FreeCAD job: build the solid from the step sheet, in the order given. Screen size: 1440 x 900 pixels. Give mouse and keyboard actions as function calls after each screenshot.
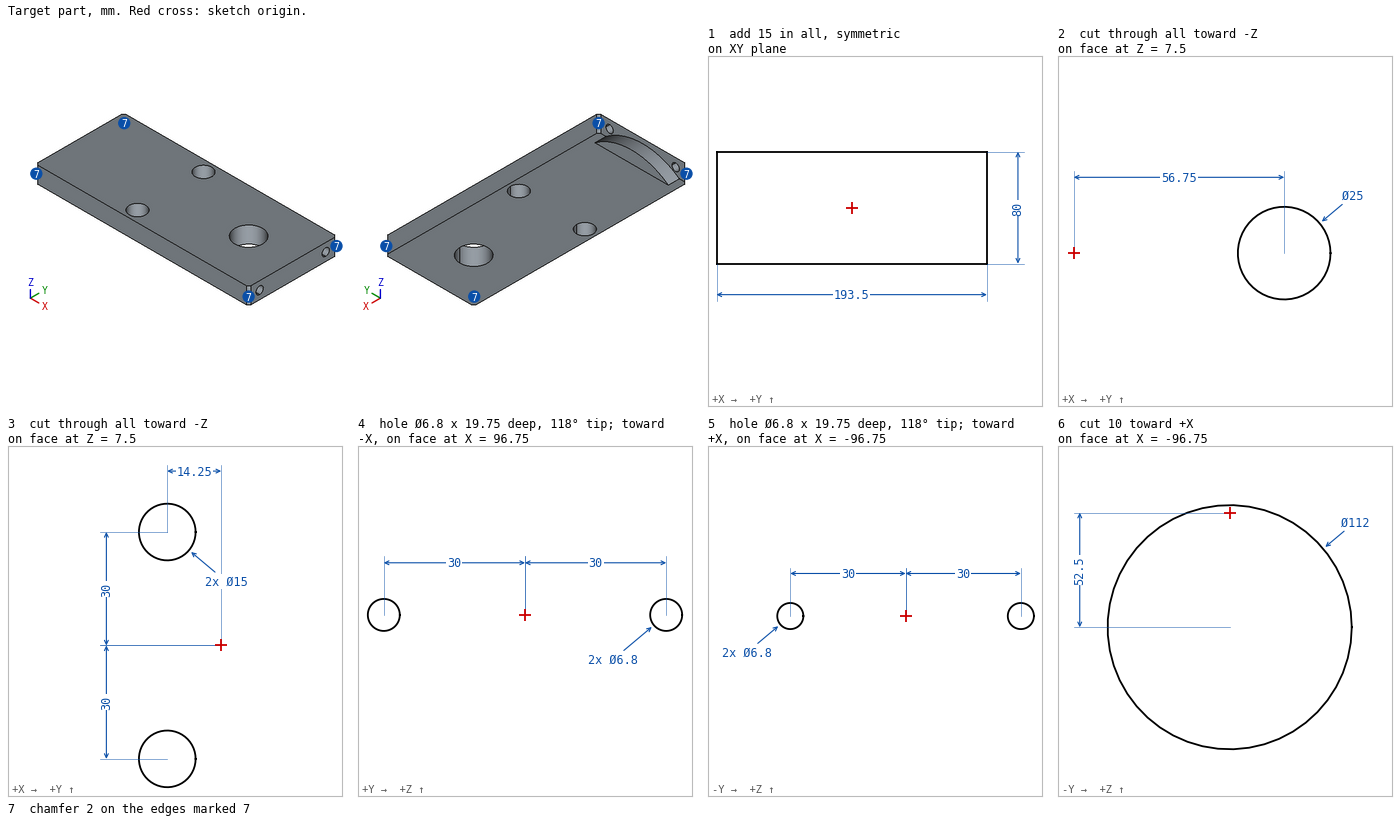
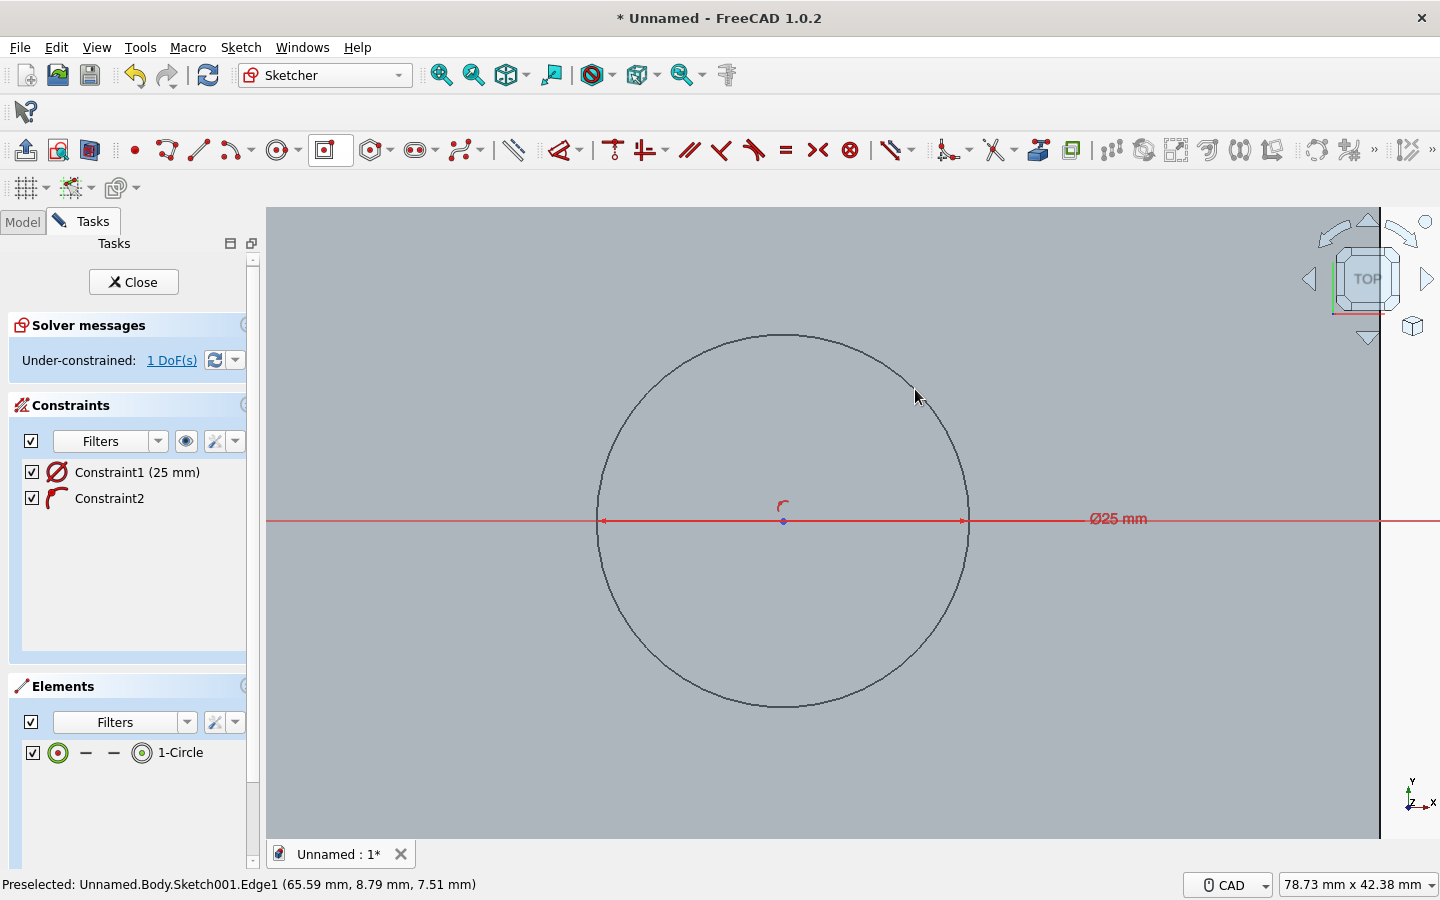
click(783, 521)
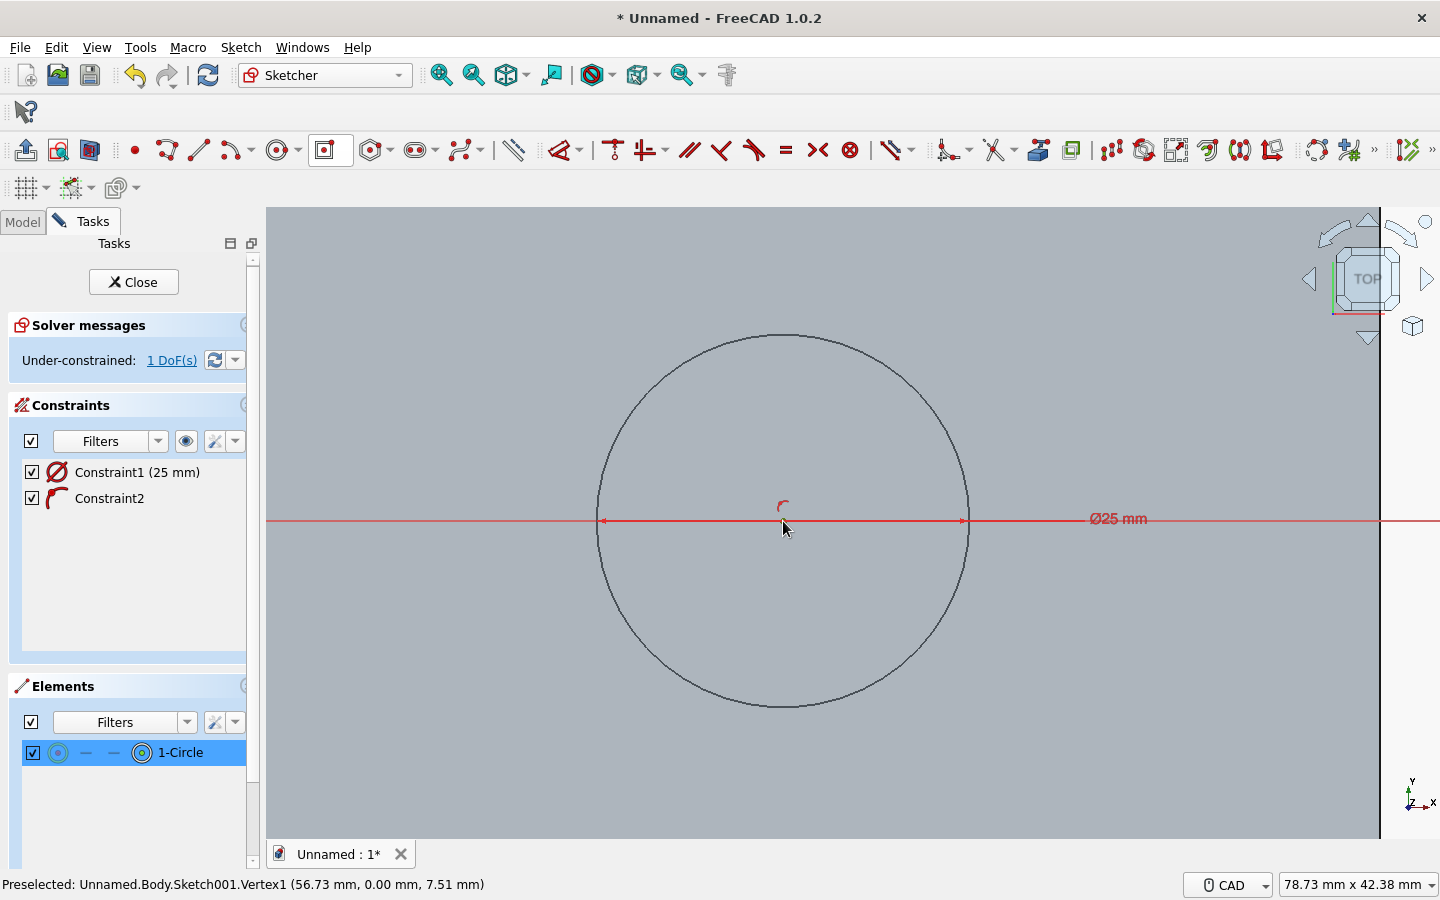
key(l)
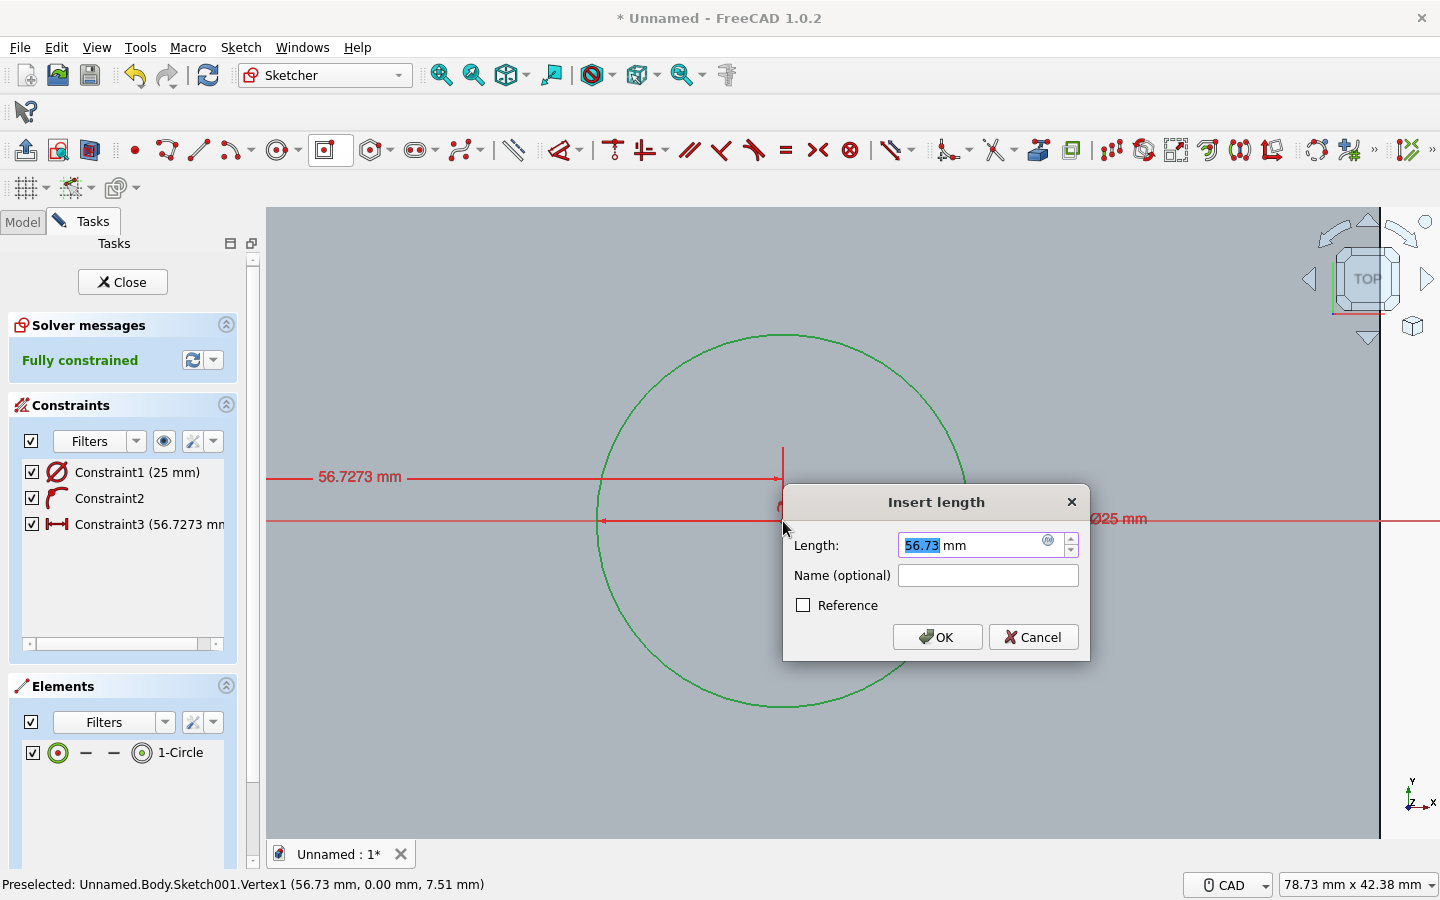
text(56.75)
key(Return)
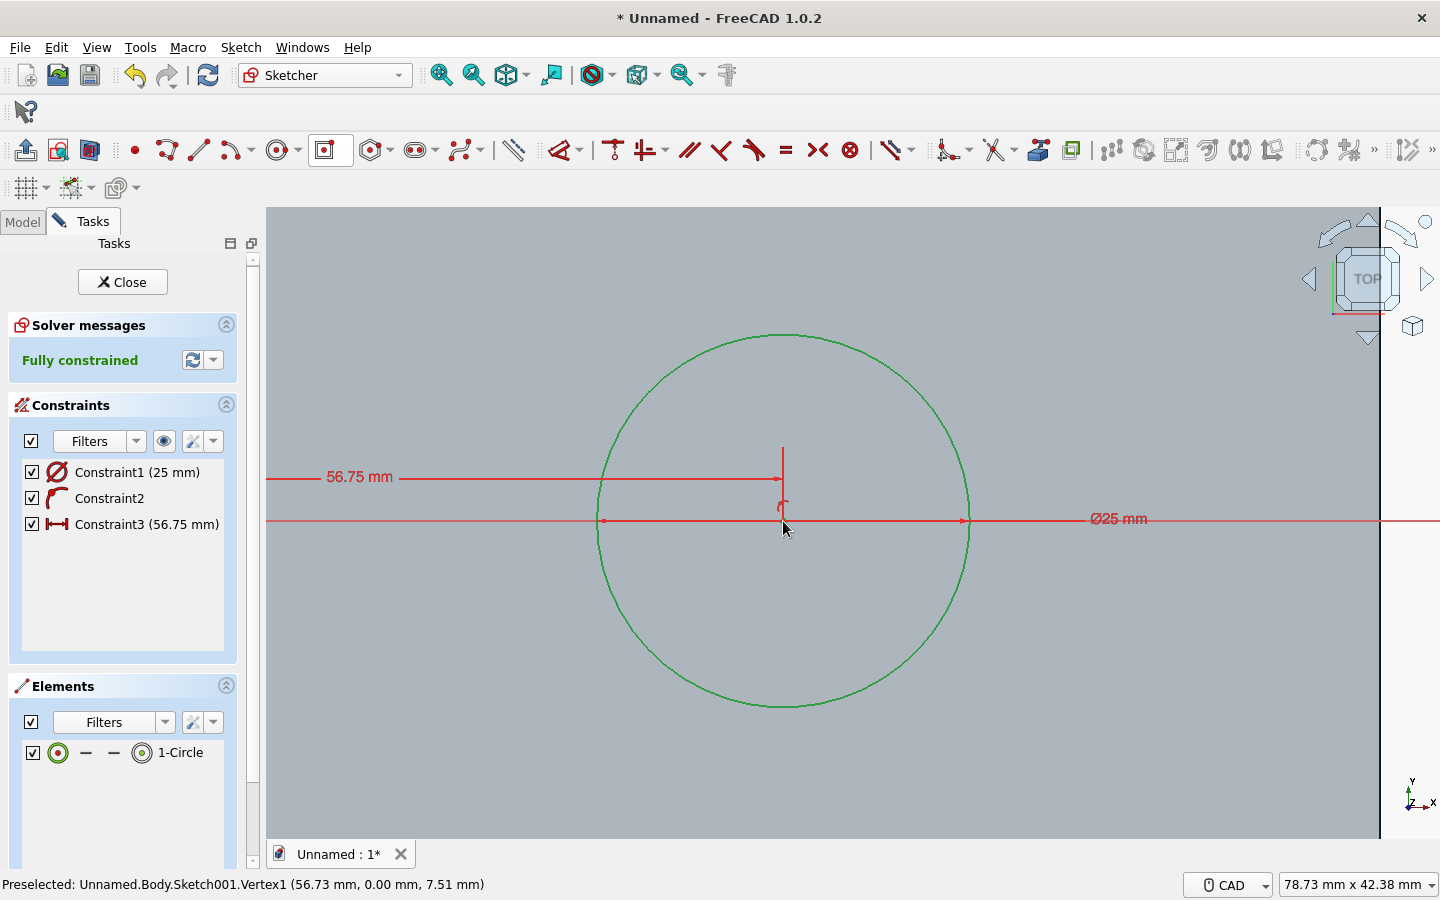
click(123, 282)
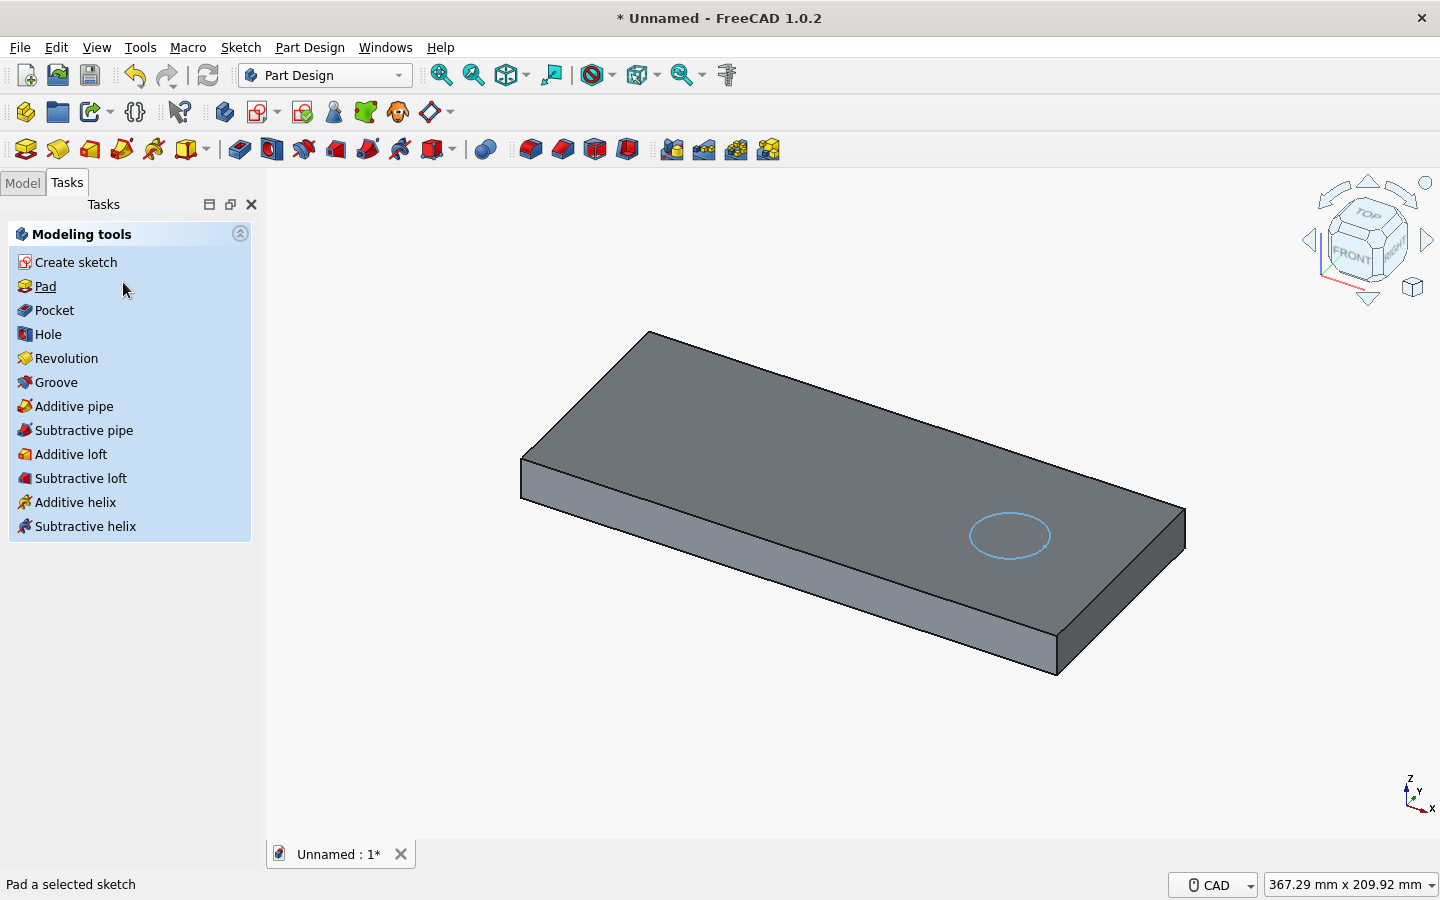
click(240, 150)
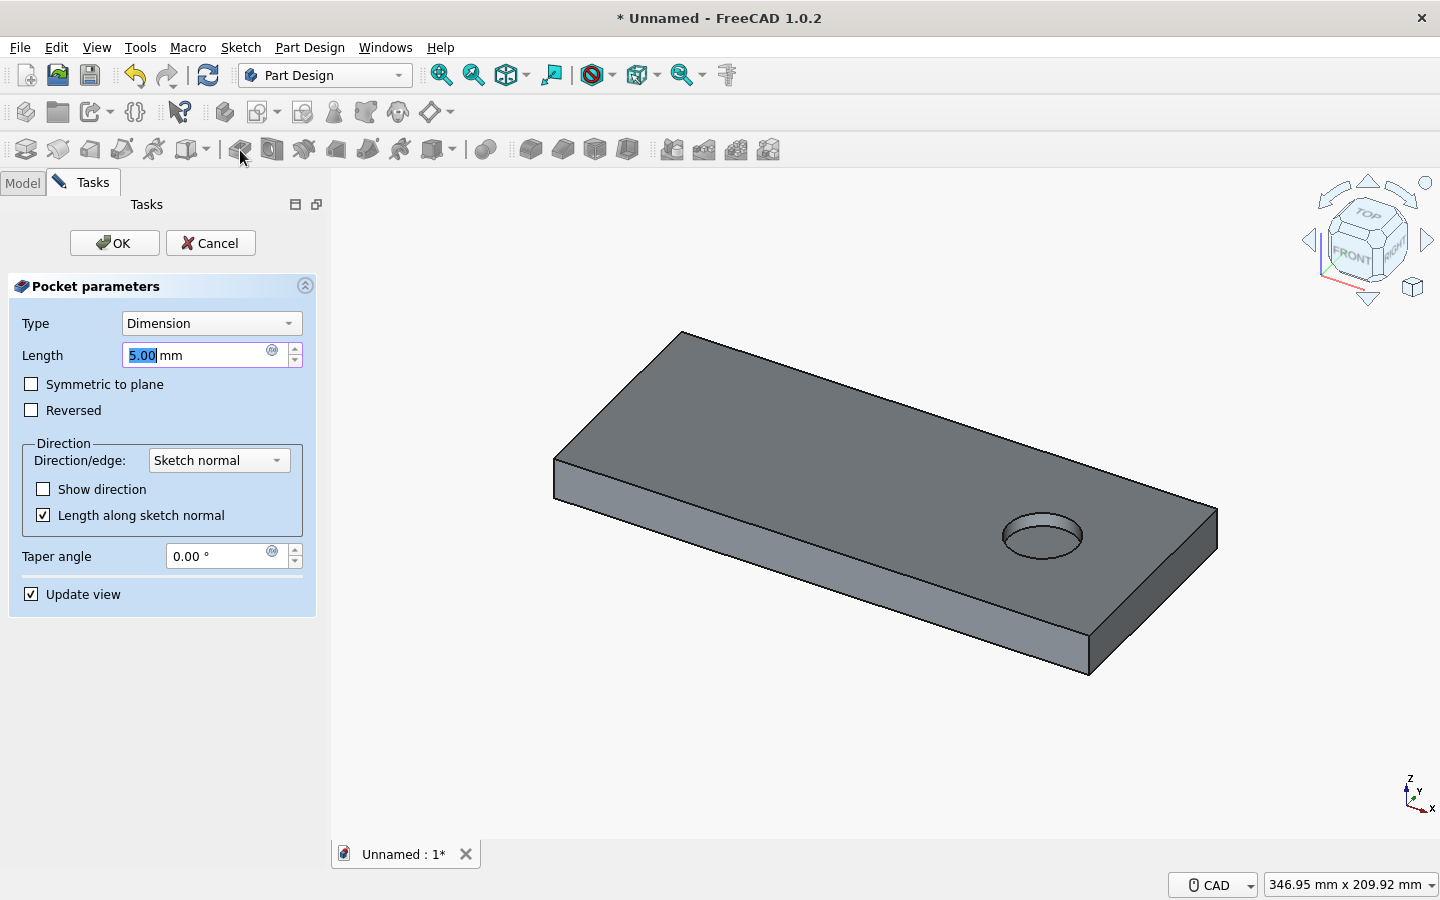
click(212, 324)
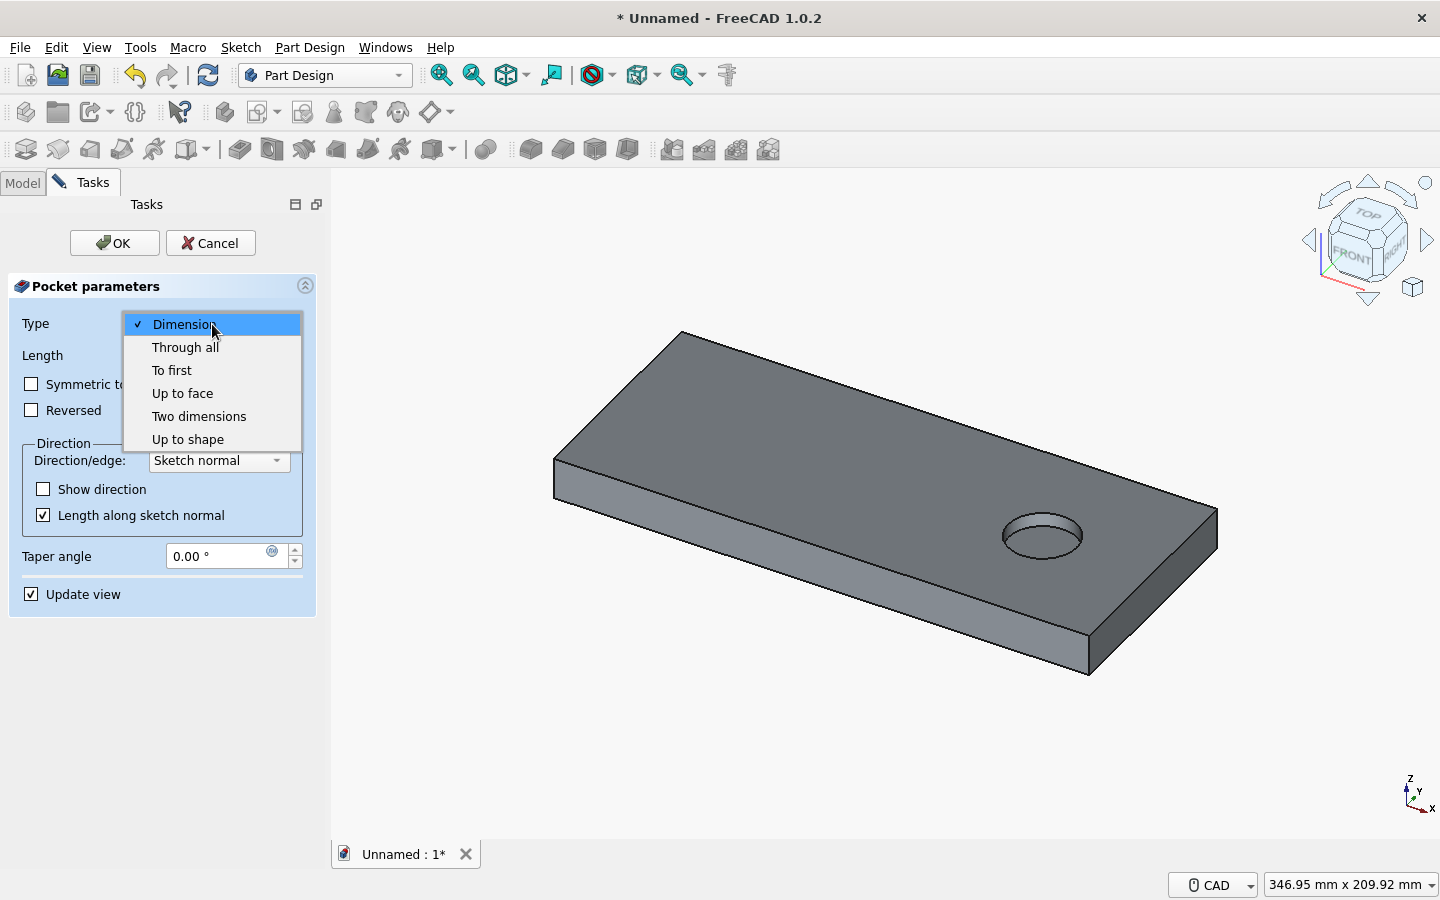
click(212, 348)